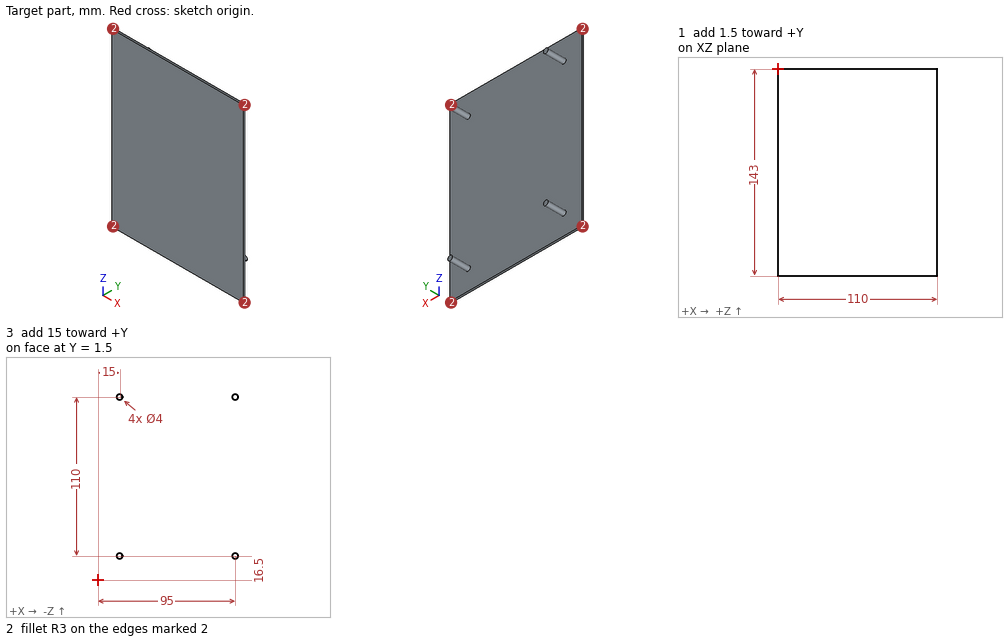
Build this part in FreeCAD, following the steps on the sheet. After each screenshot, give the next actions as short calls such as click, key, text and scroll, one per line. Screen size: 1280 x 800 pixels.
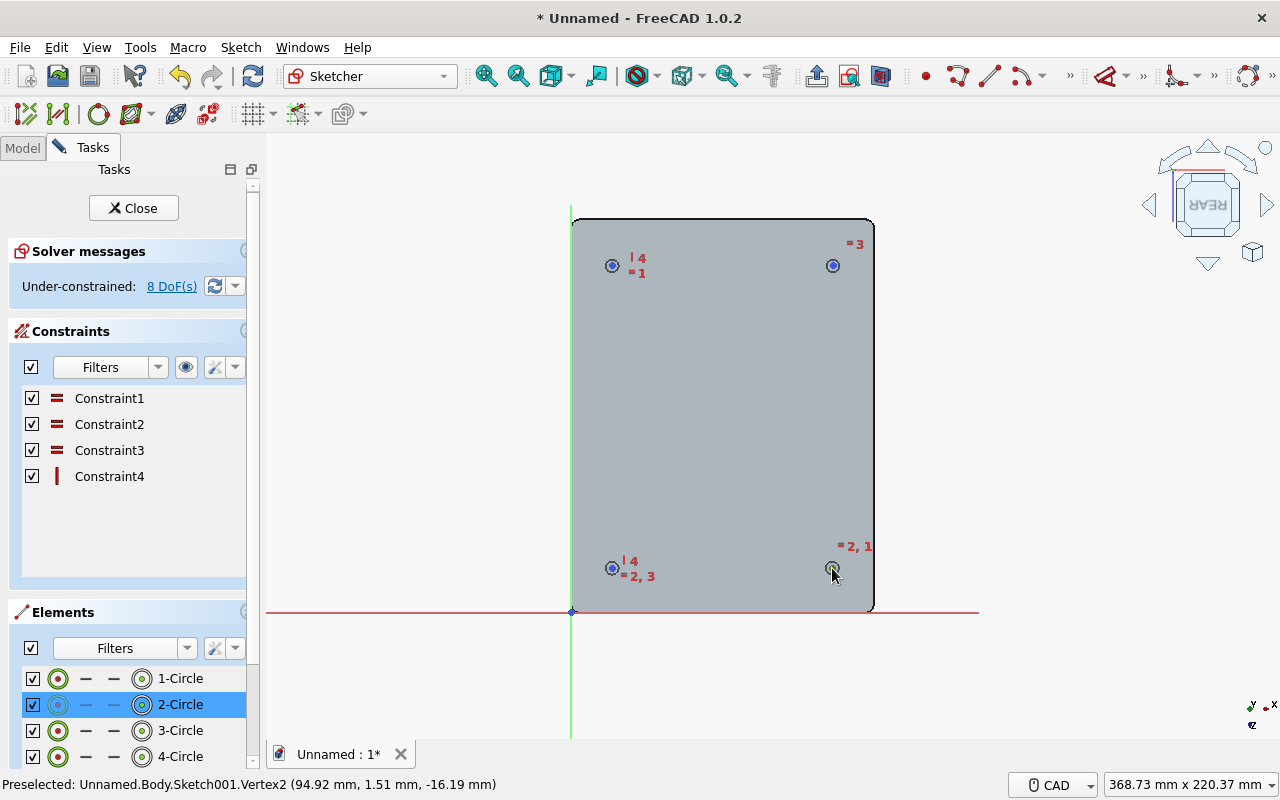
click(612, 568)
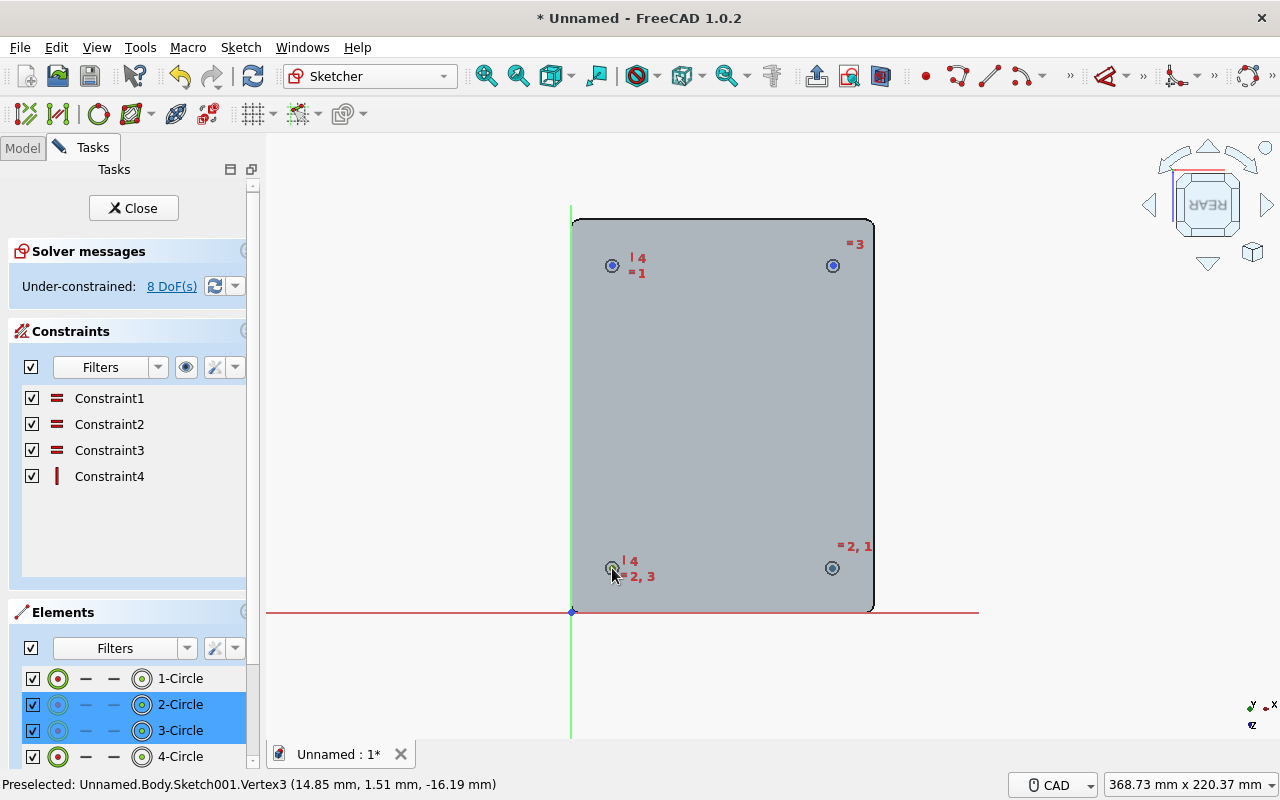
key(h)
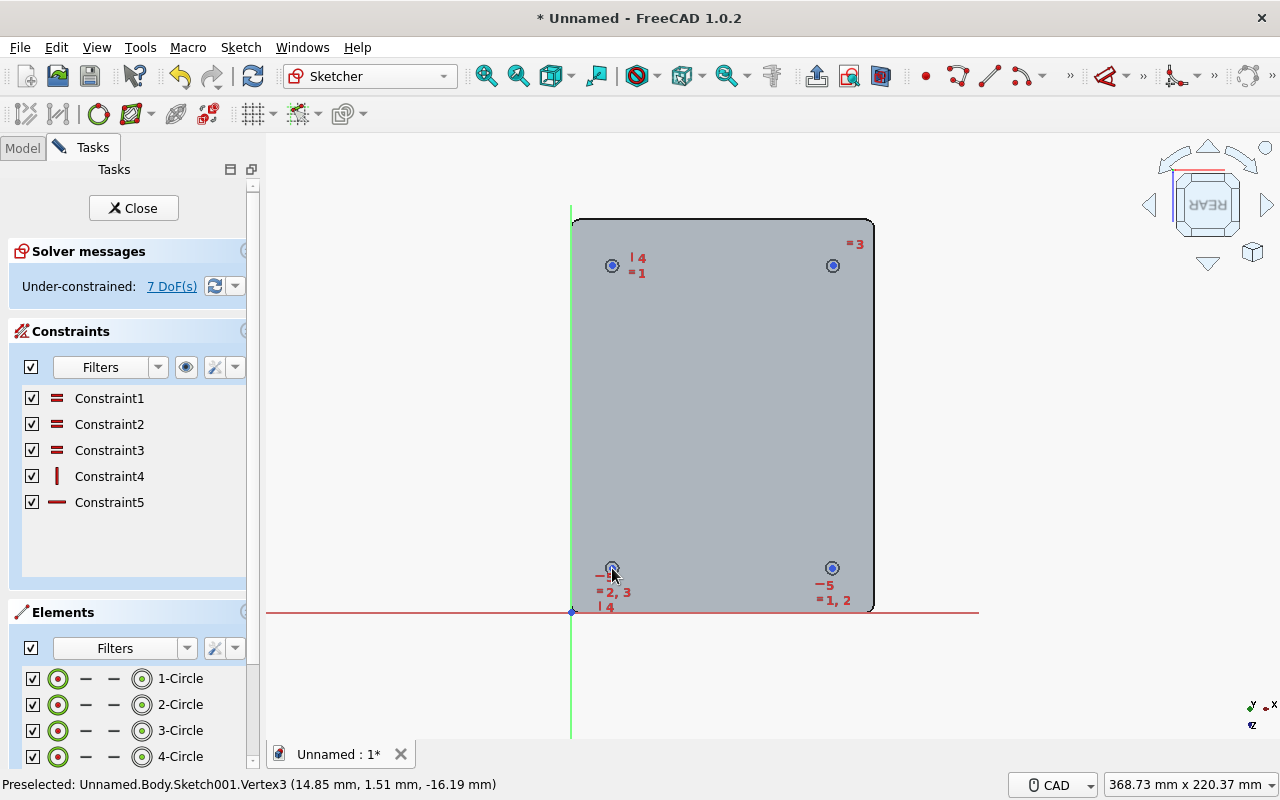
click(832, 568)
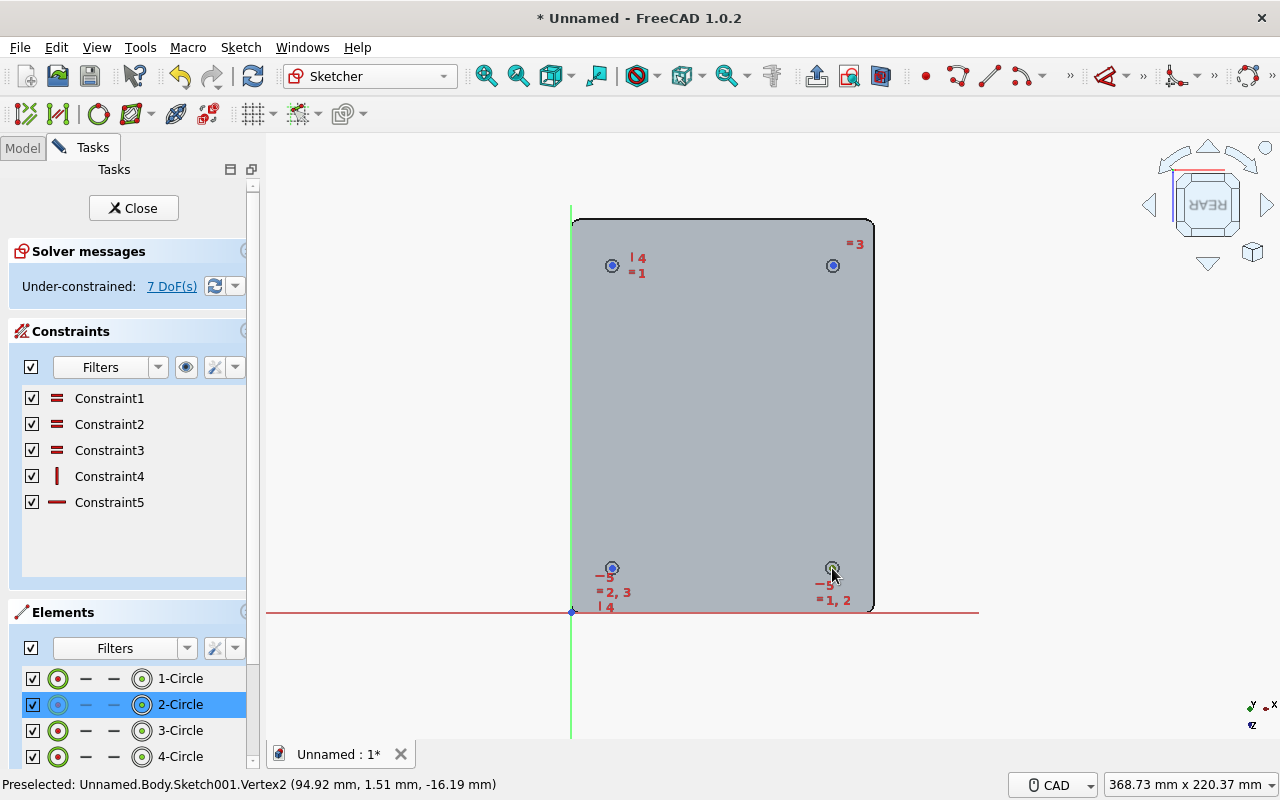
click(833, 266)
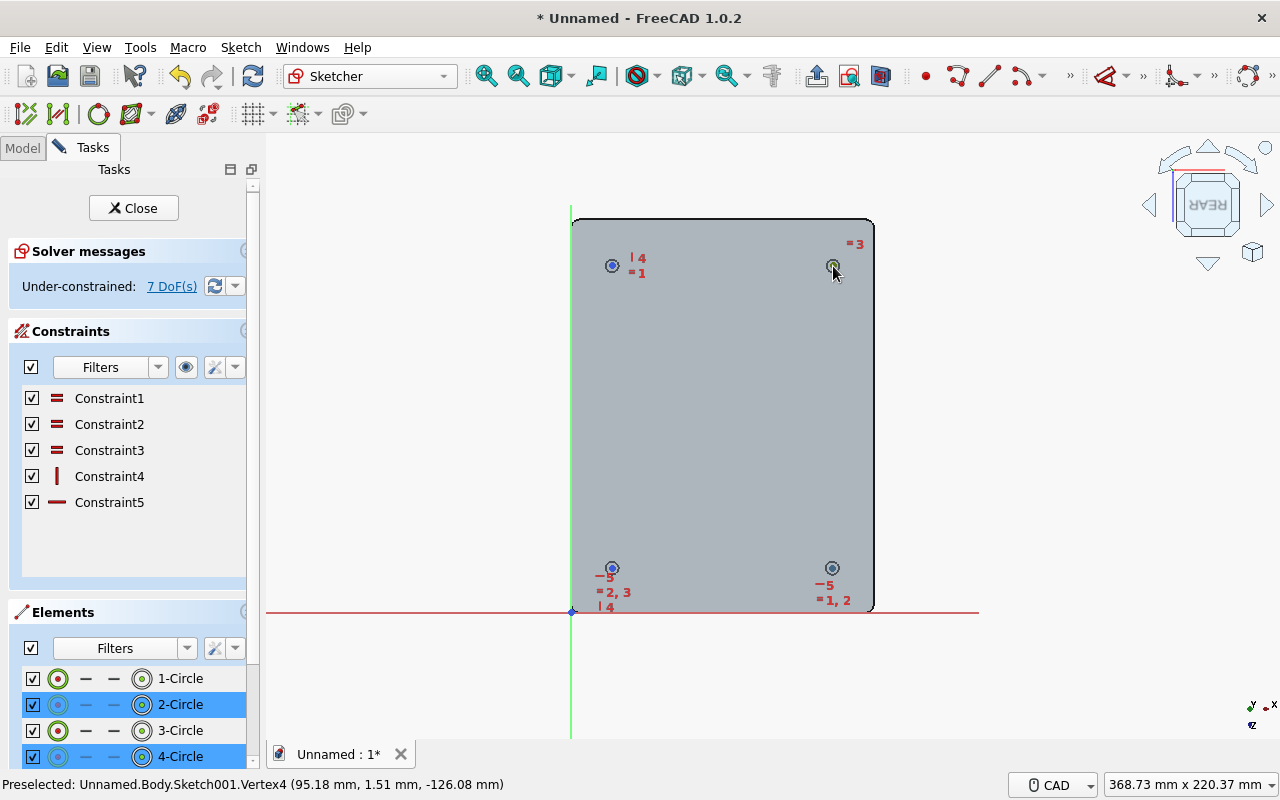
key(v)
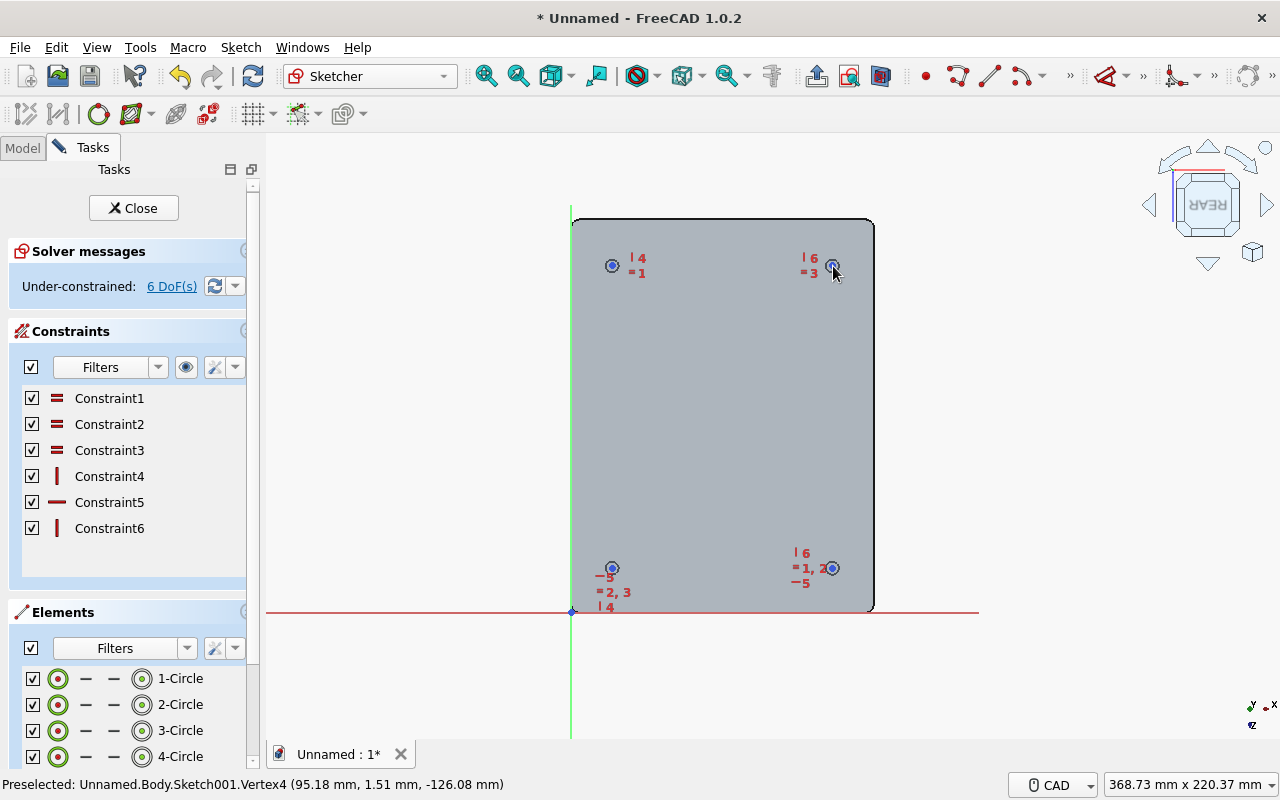
click(612, 266)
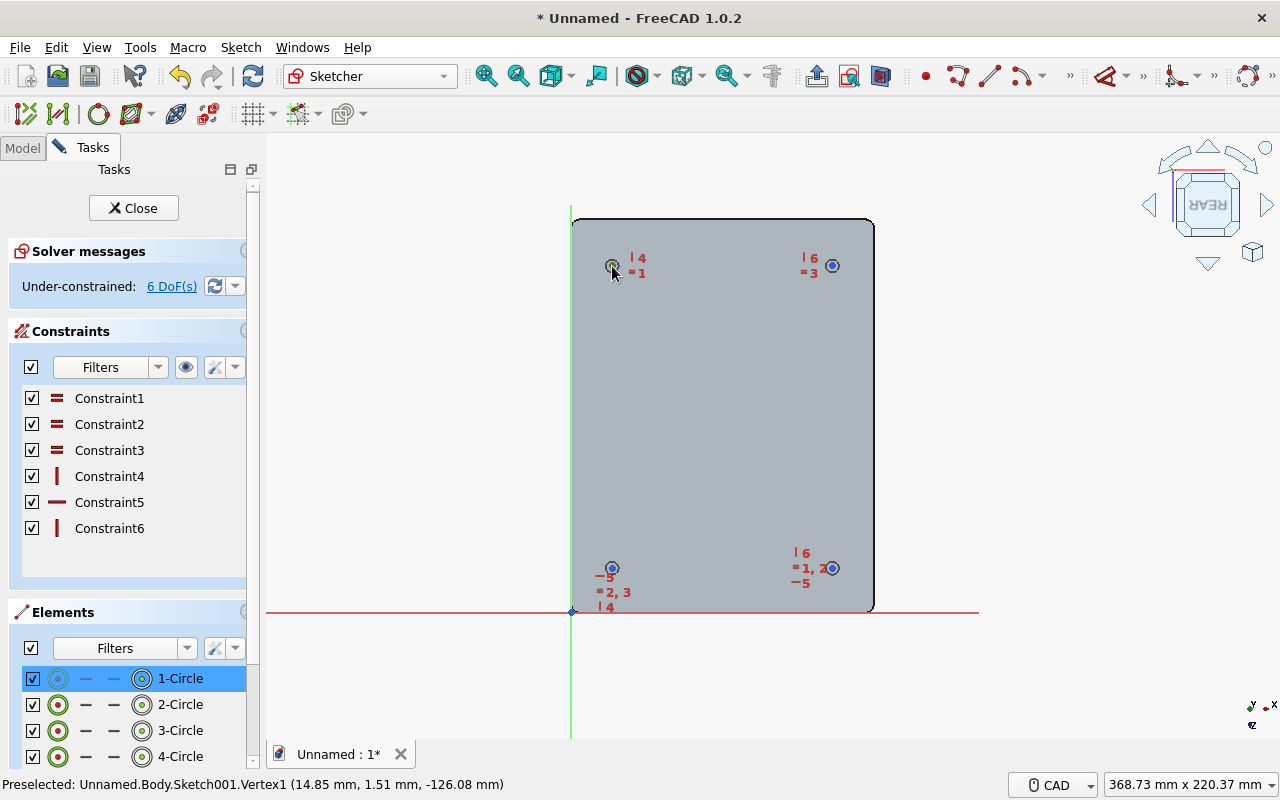
click(832, 266)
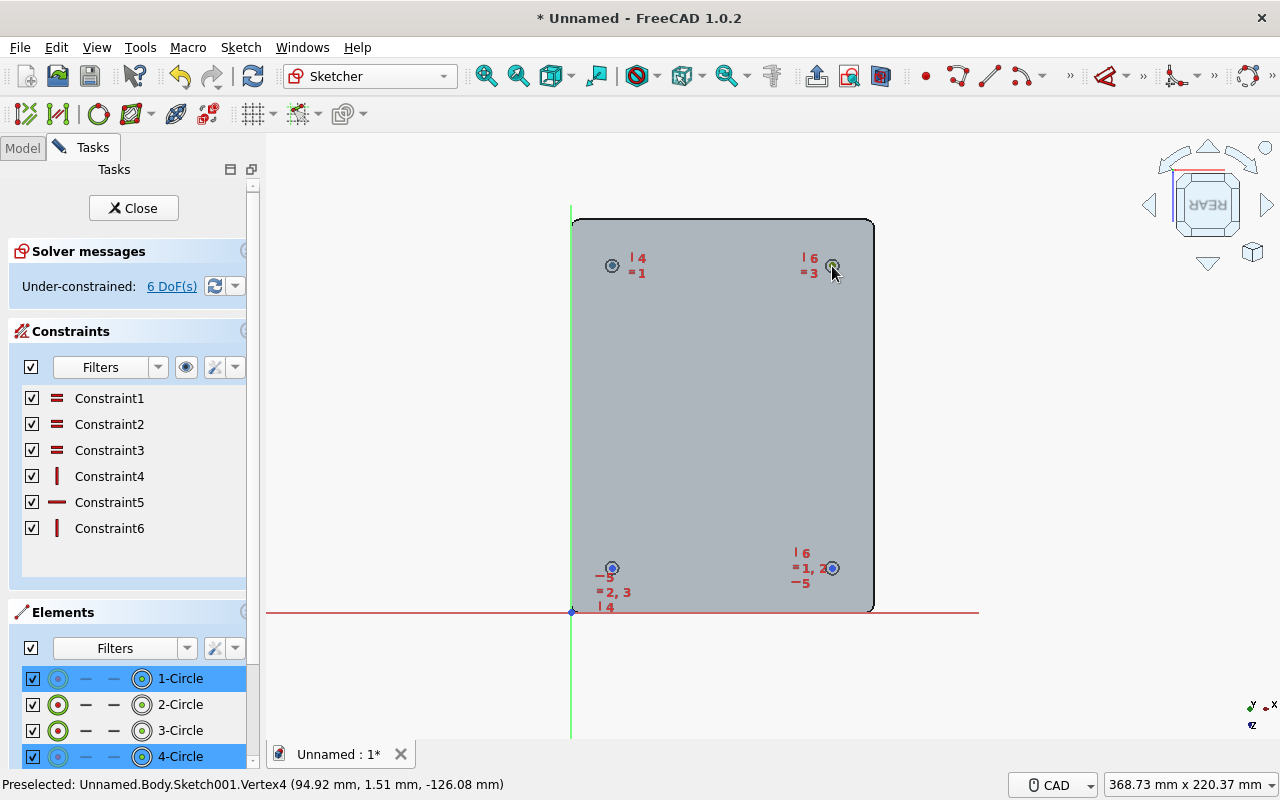
key(h)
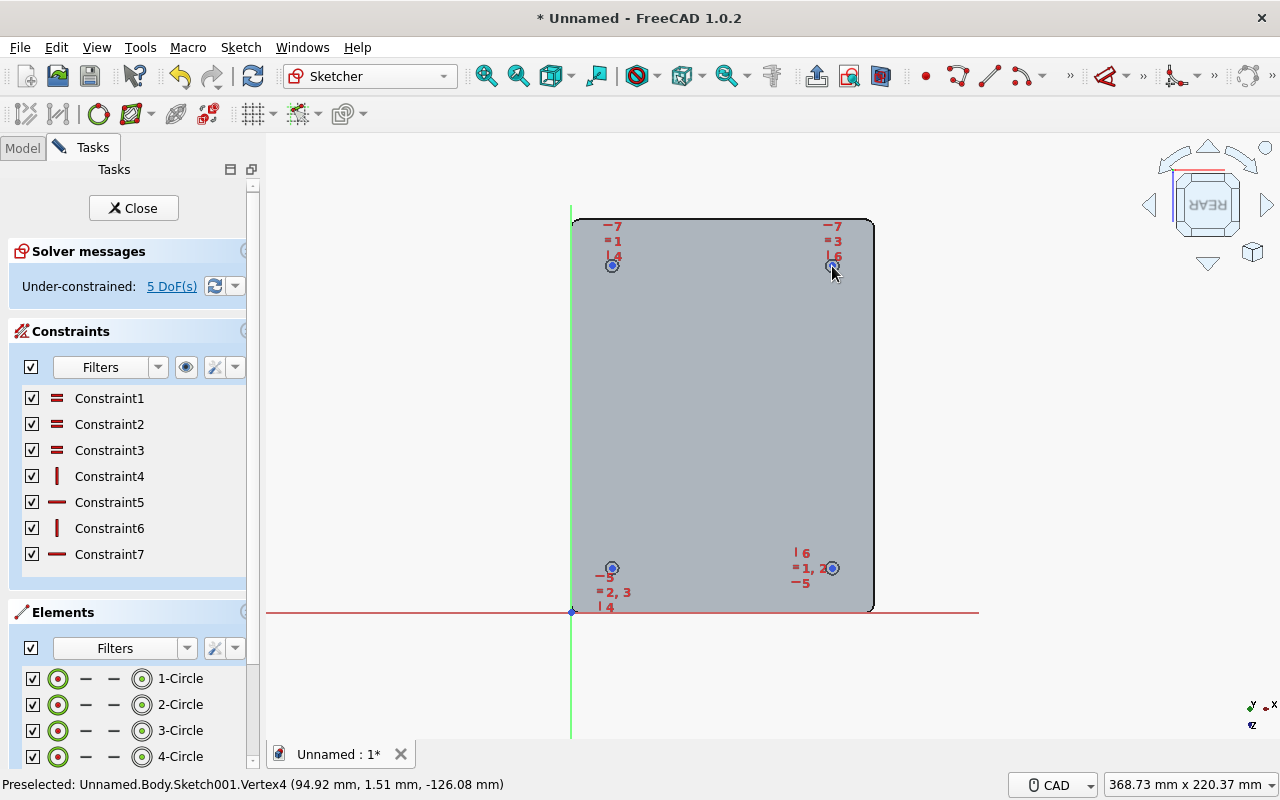
click(1106, 76)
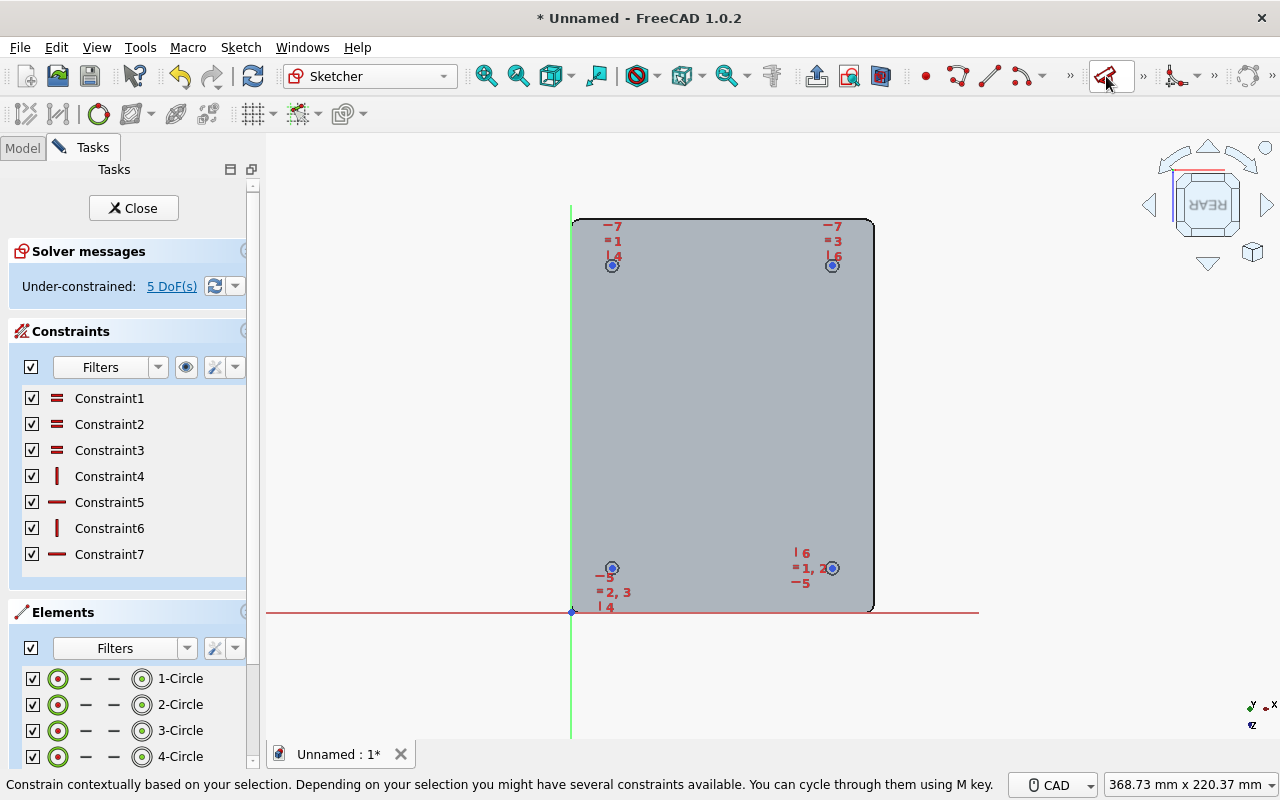
scroll(617, 261, up, 7)